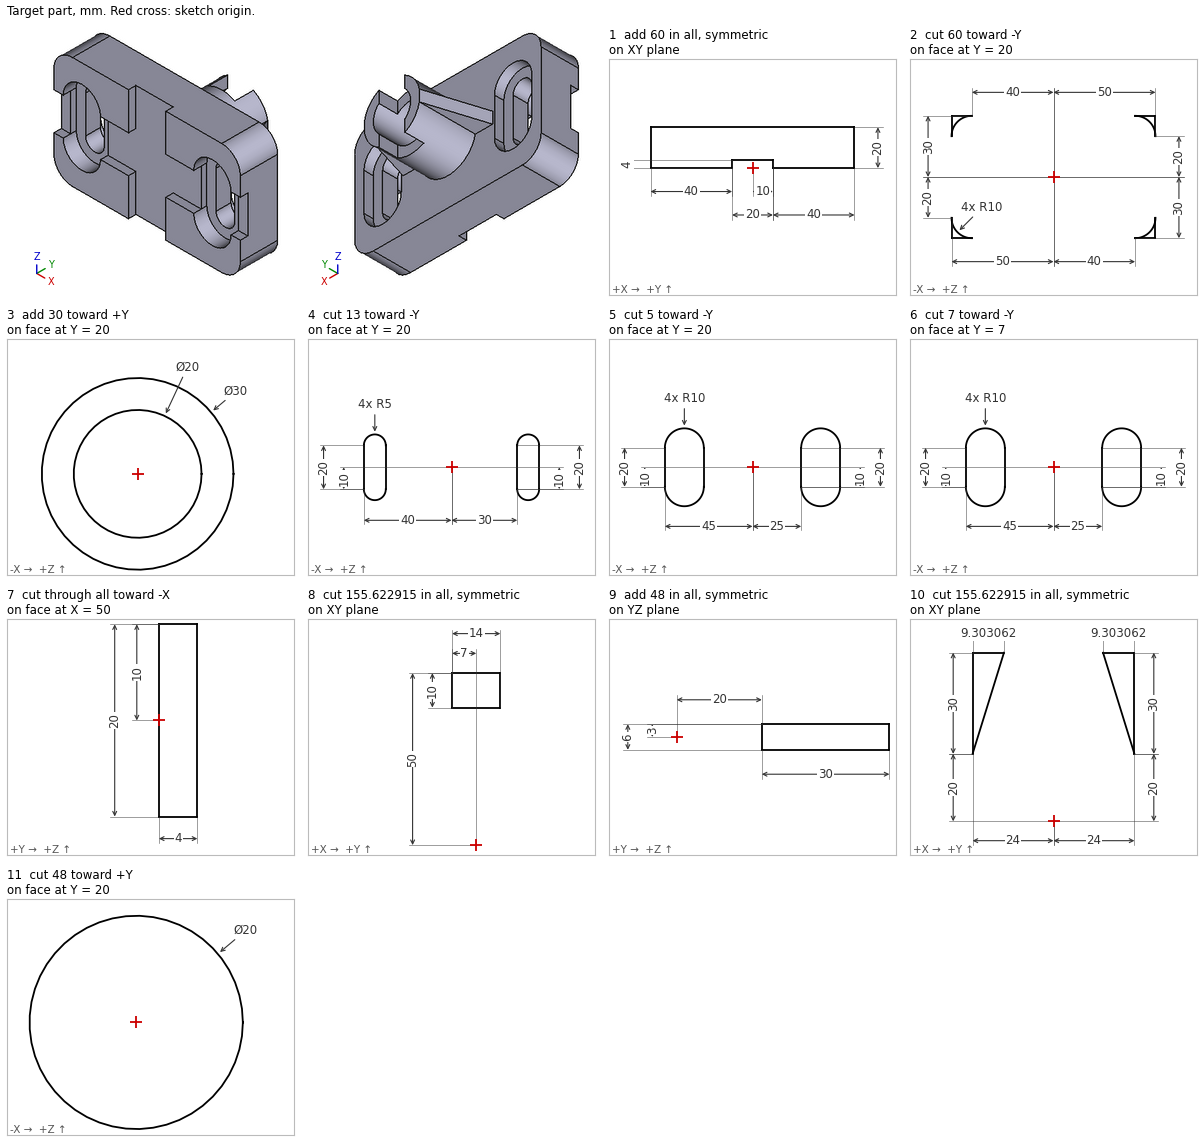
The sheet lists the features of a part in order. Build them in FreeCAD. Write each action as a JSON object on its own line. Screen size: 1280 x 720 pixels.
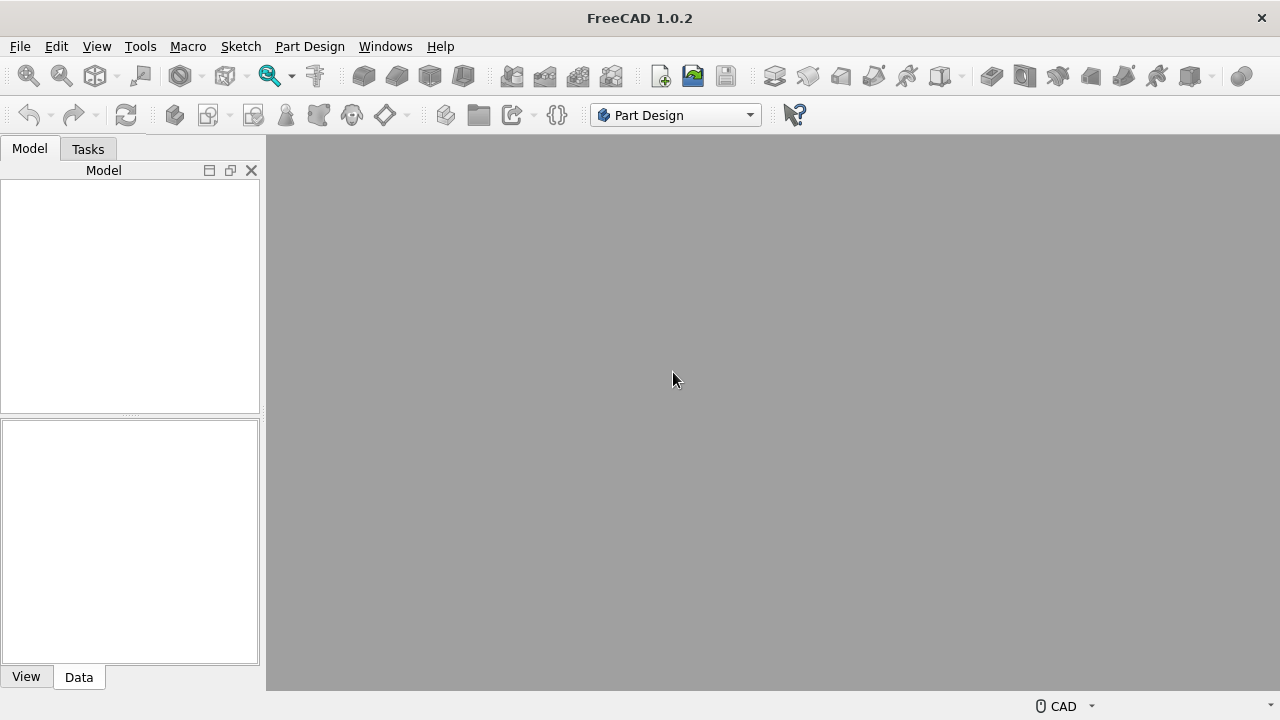
{"action": "key", "text": "ctrl+n"}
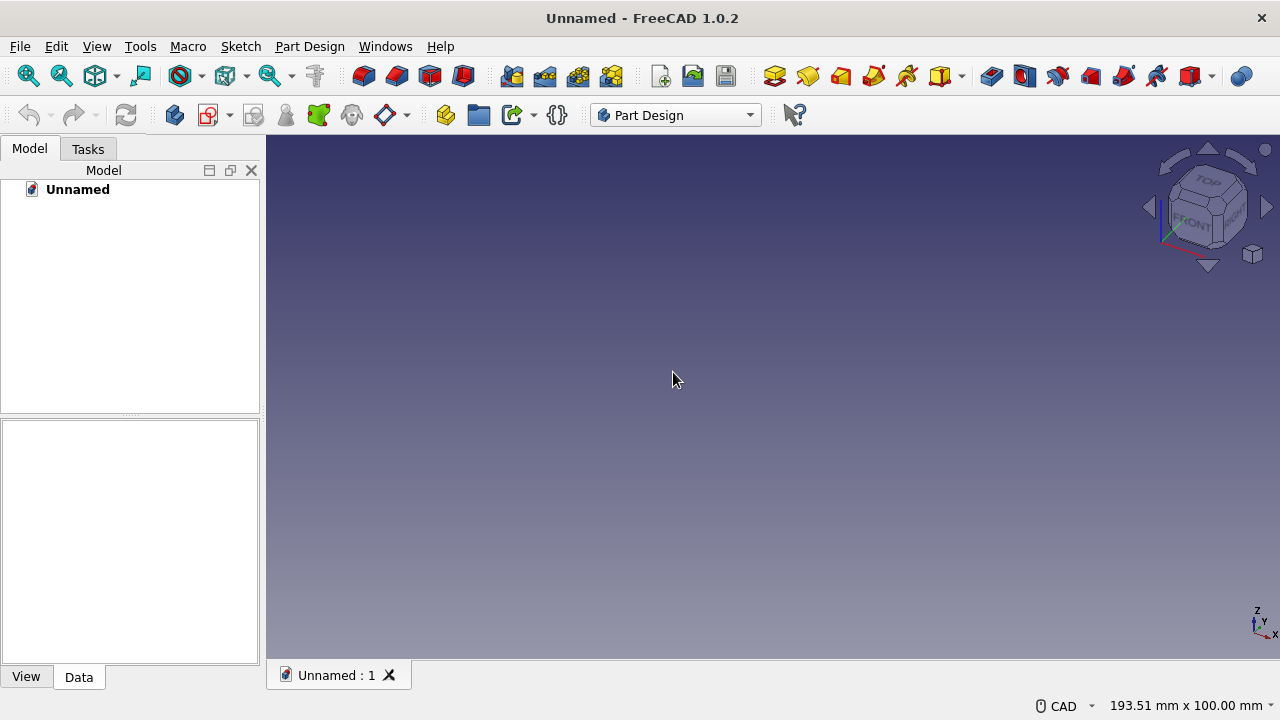
{"action": "left_click", "coordinate": [208, 116]}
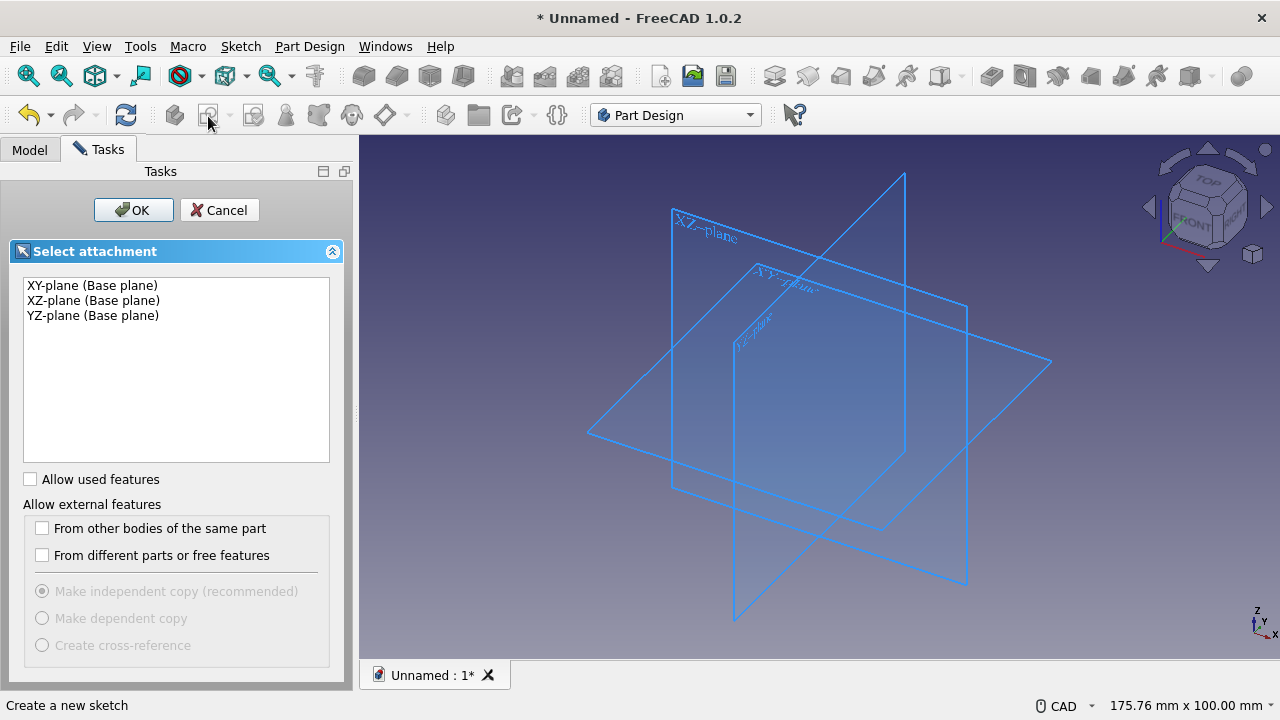
{"action": "left_click", "coordinate": [84, 286]}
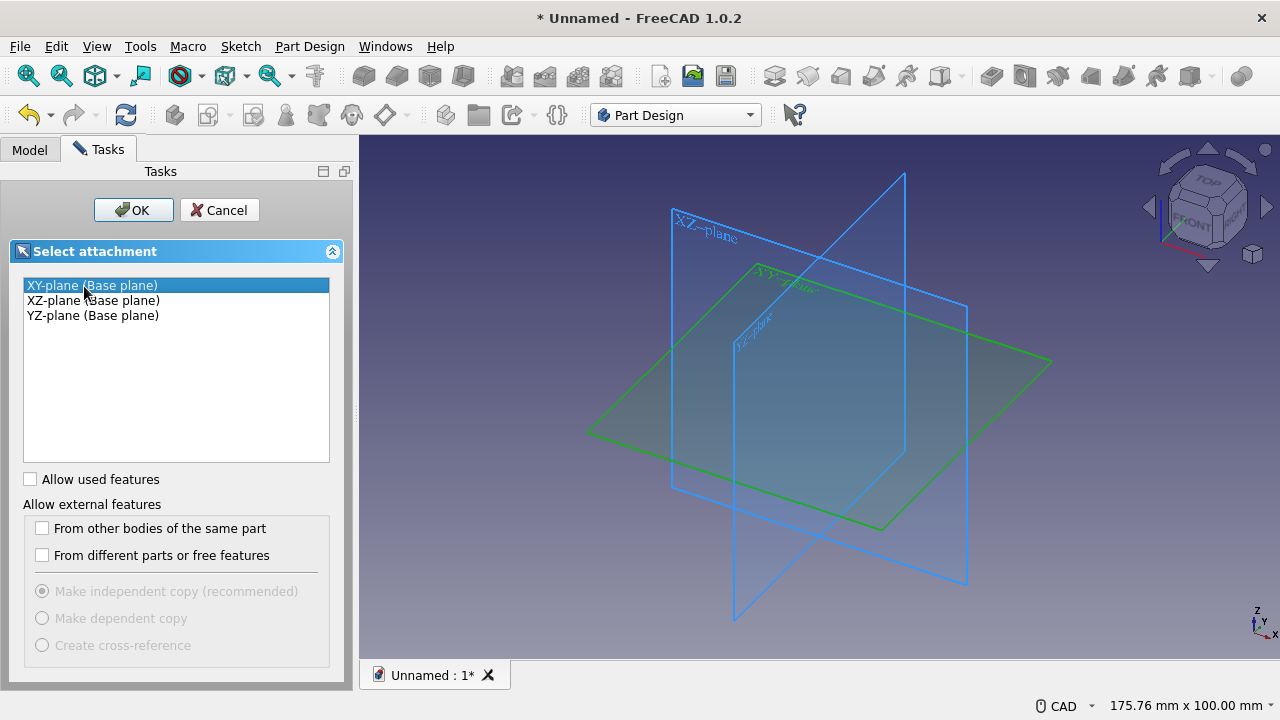
{"action": "left_click", "coordinate": [134, 210]}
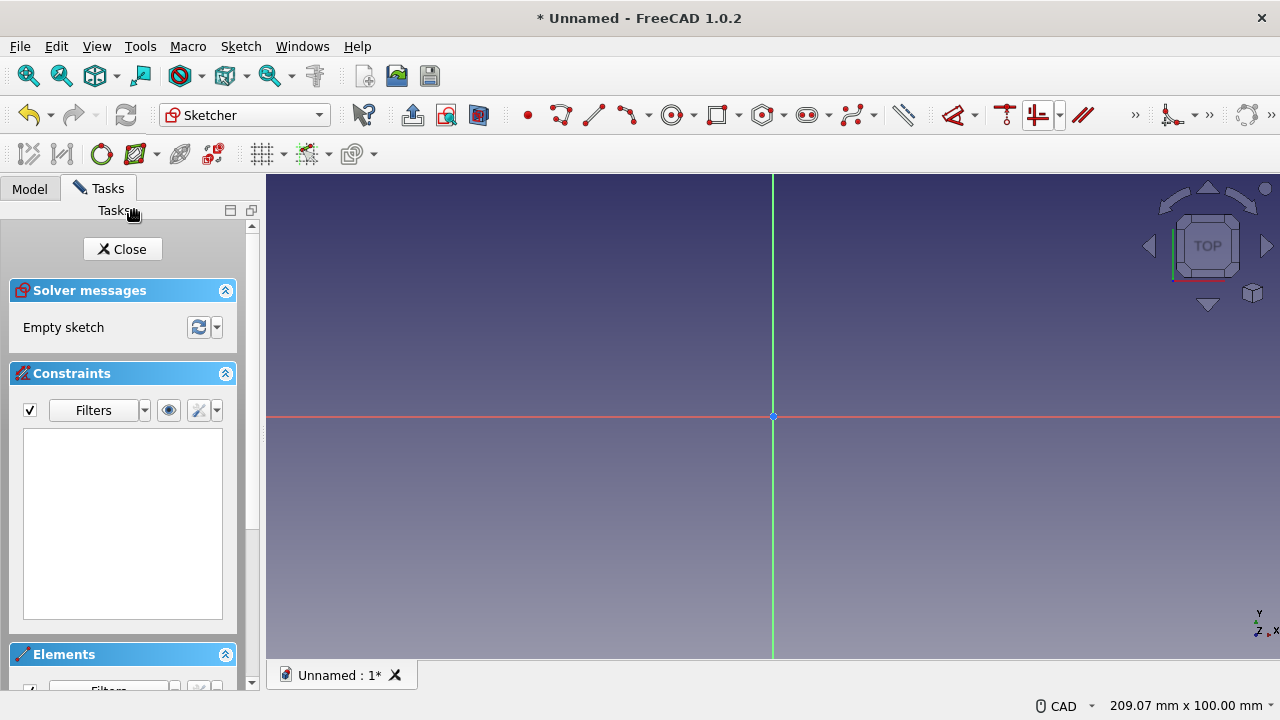
{"action": "key", "text": "g m"}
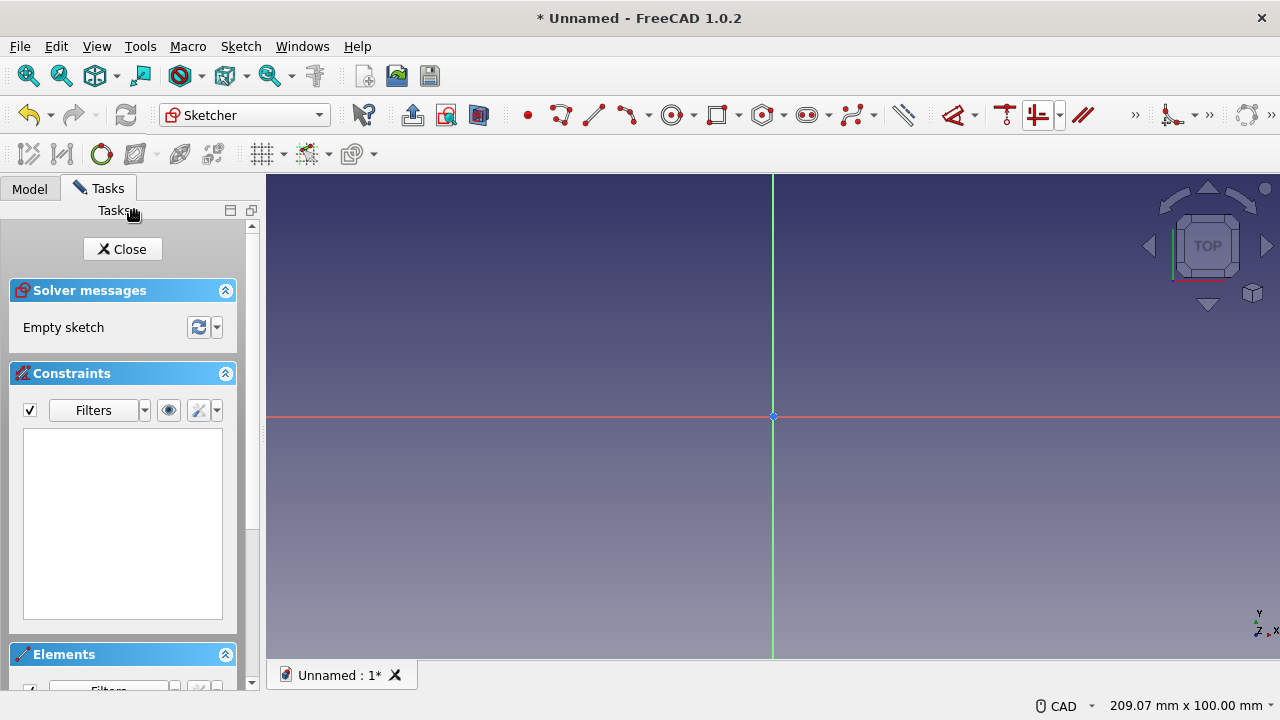
{"action": "left_click", "coordinate": [822, 416]}
{"action": "left_click", "coordinate": [1016, 408]}
{"action": "left_click", "coordinate": [1016, 320]}
{"action": "left_click", "coordinate": [530, 320]}
{"action": "left_click", "coordinate": [530, 416]}
{"action": "left_click", "coordinate": [724, 408]}
{"action": "left_click", "coordinate": [724, 397]}
{"action": "left_click", "coordinate": [822, 397]}
{"action": "left_click", "coordinate": [822, 416]}
{"action": "key", "text": "Escape"}
{"action": "key", "text": "Escape"}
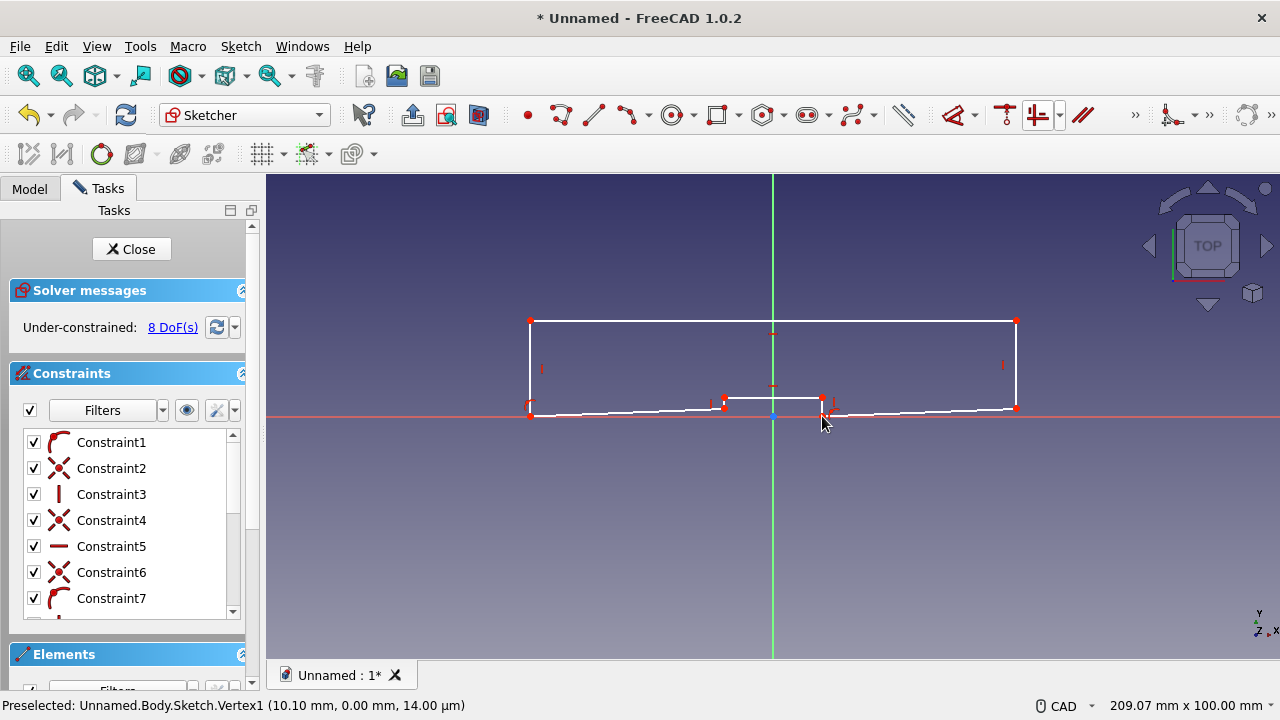
{"action": "left_click", "coordinate": [880, 414]}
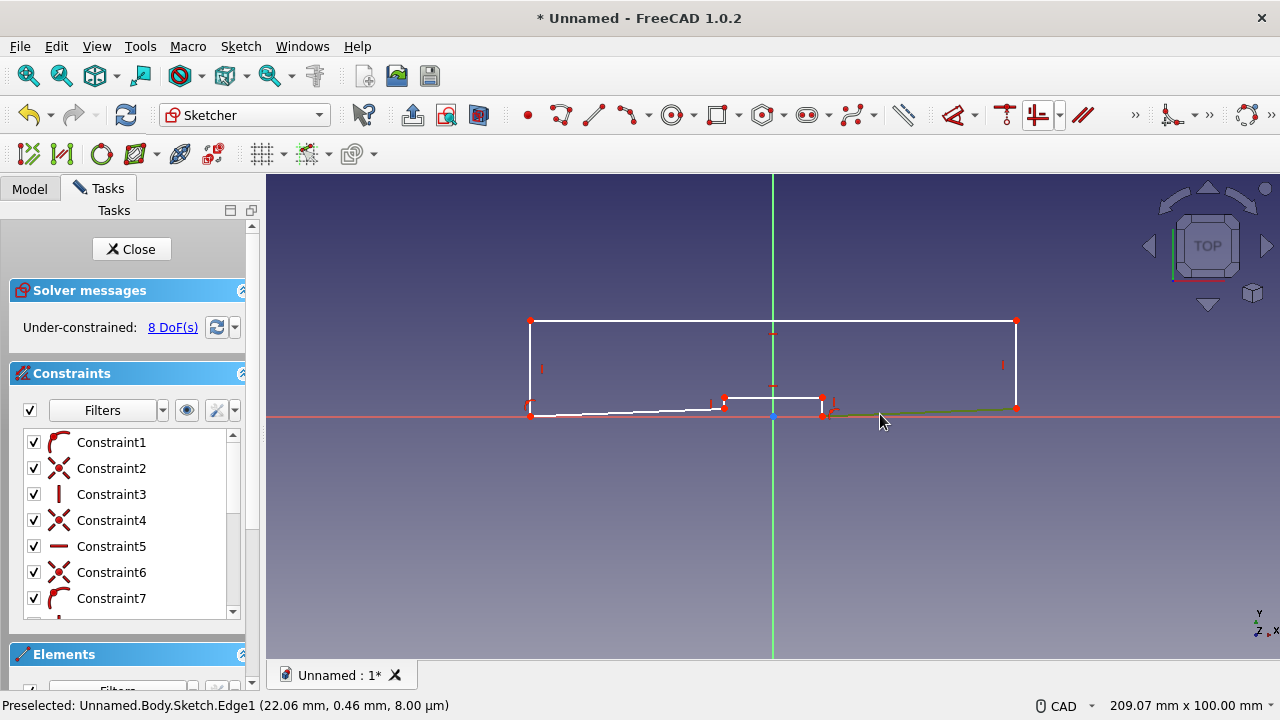
{"action": "key", "text": "h"}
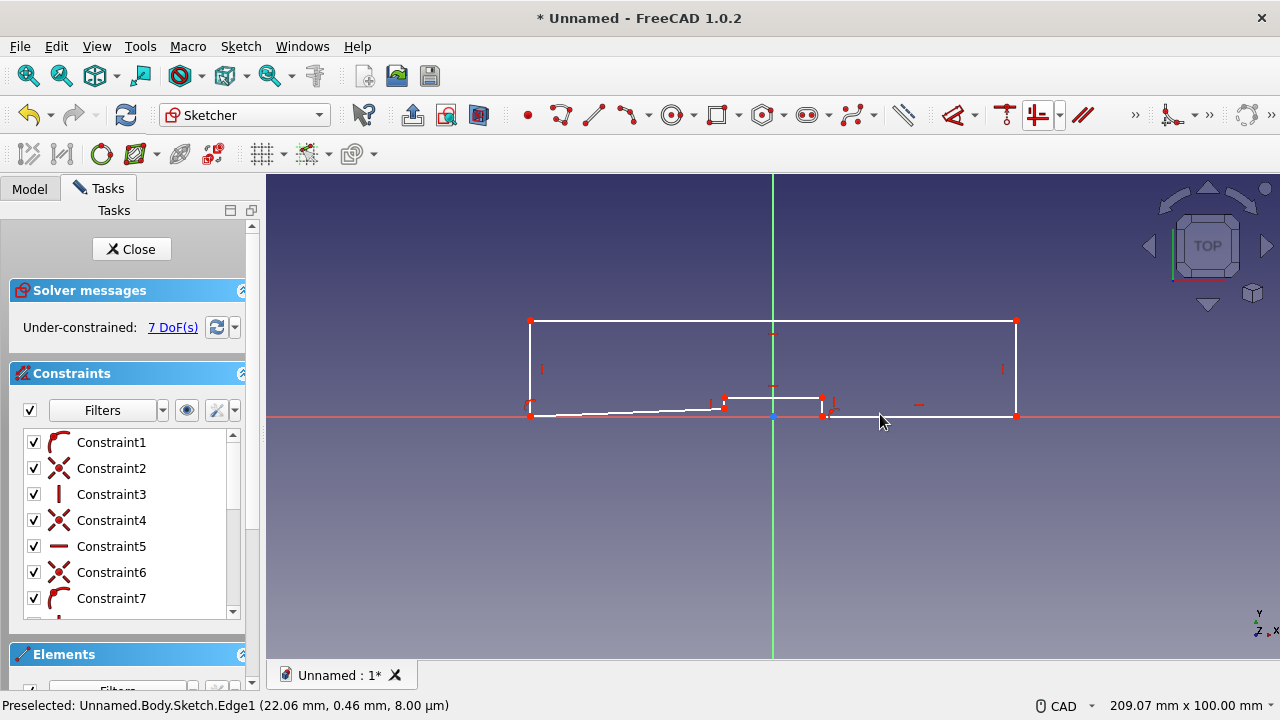
{"action": "left_click", "coordinate": [588, 414]}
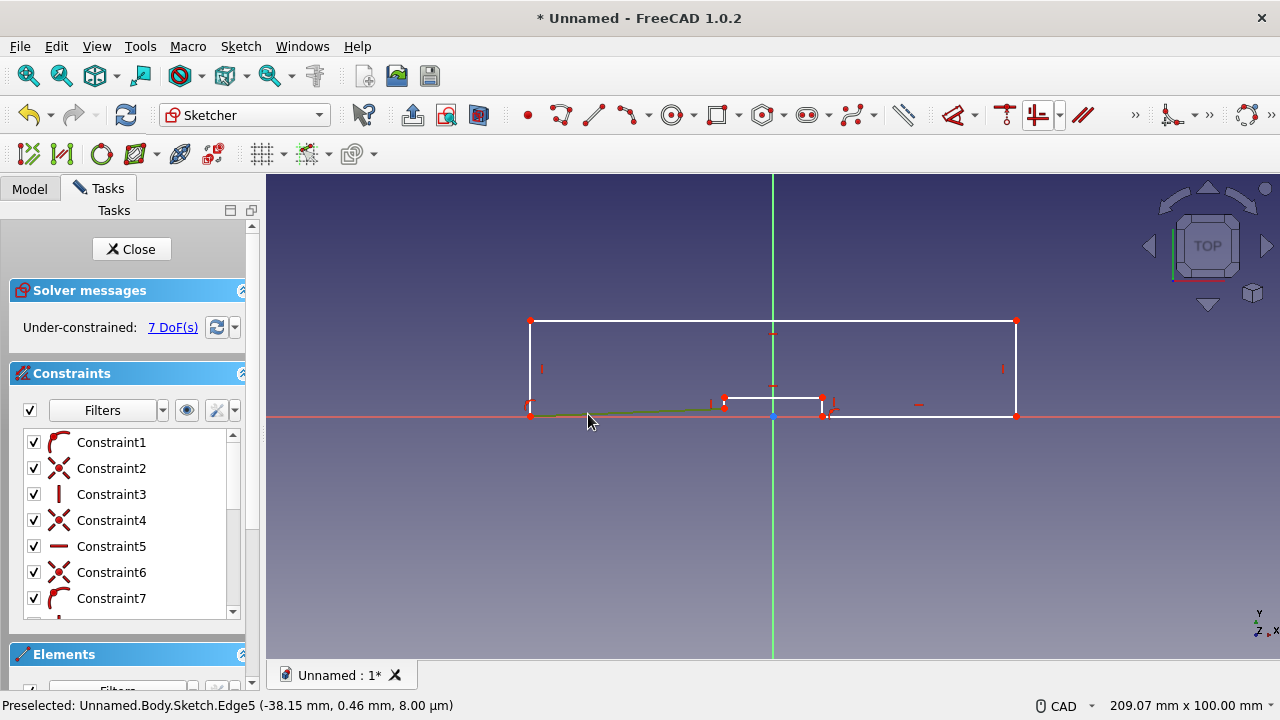
{"action": "left_click", "coordinate": [1060, 116]}